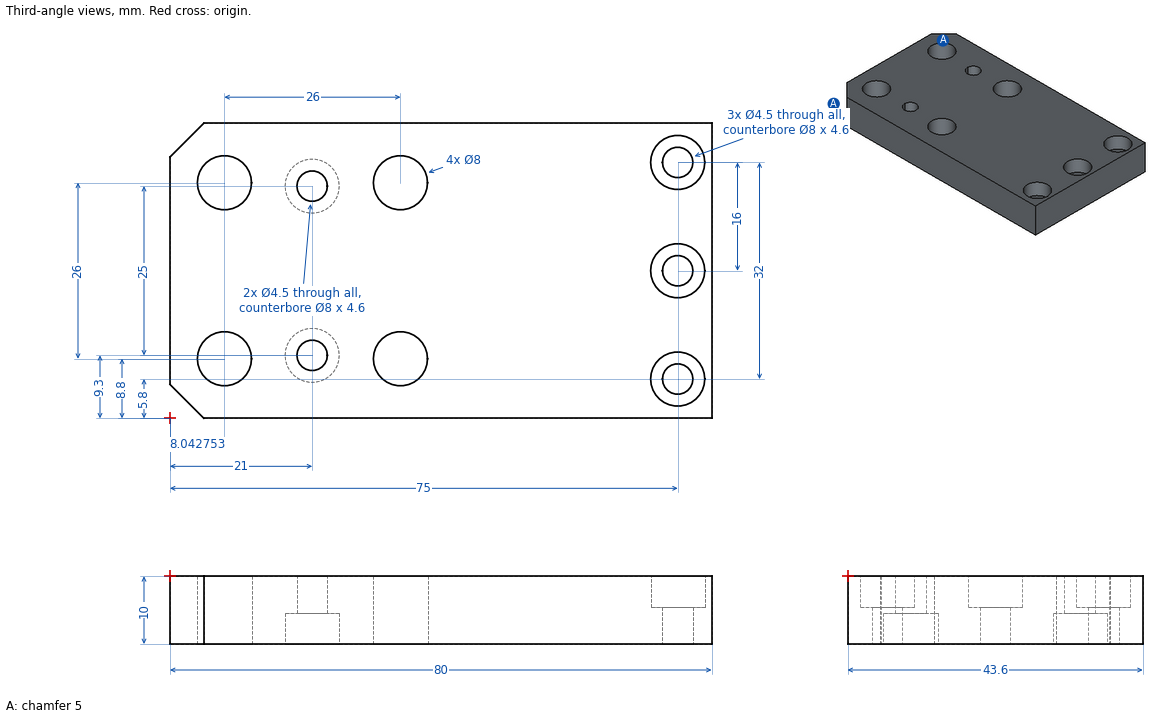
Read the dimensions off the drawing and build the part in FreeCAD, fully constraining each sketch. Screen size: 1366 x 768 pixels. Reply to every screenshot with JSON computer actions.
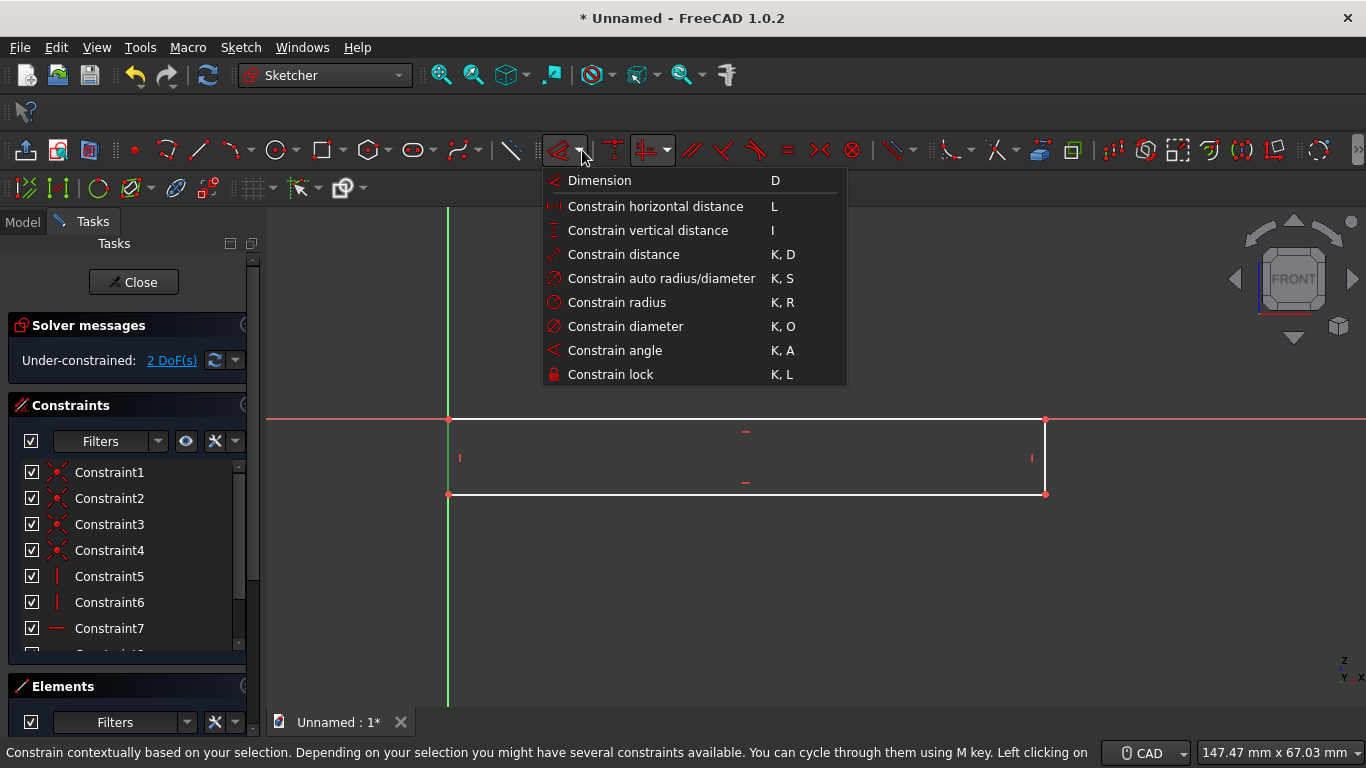
{"action": "left_click", "coordinate": [695, 230]}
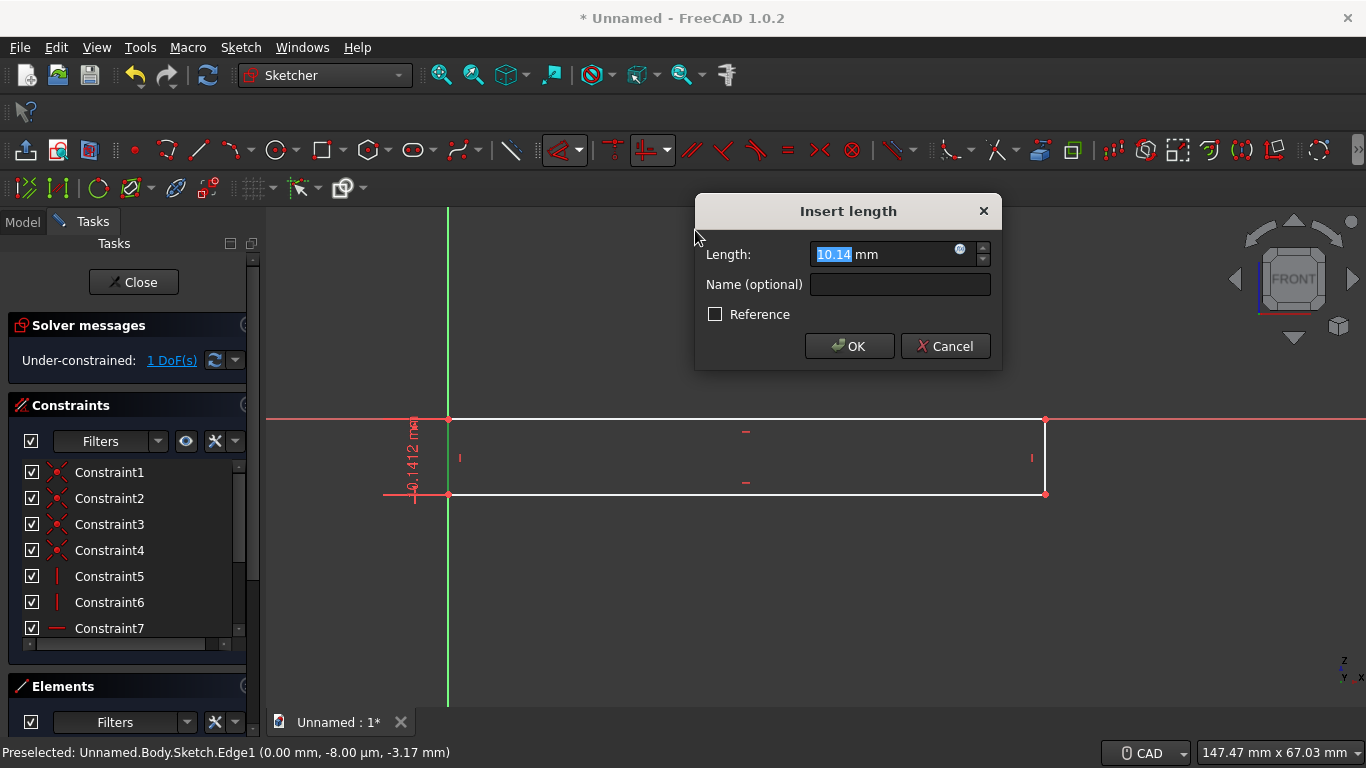
{"action": "type", "text": "10"}
{"action": "key", "text": "Return"}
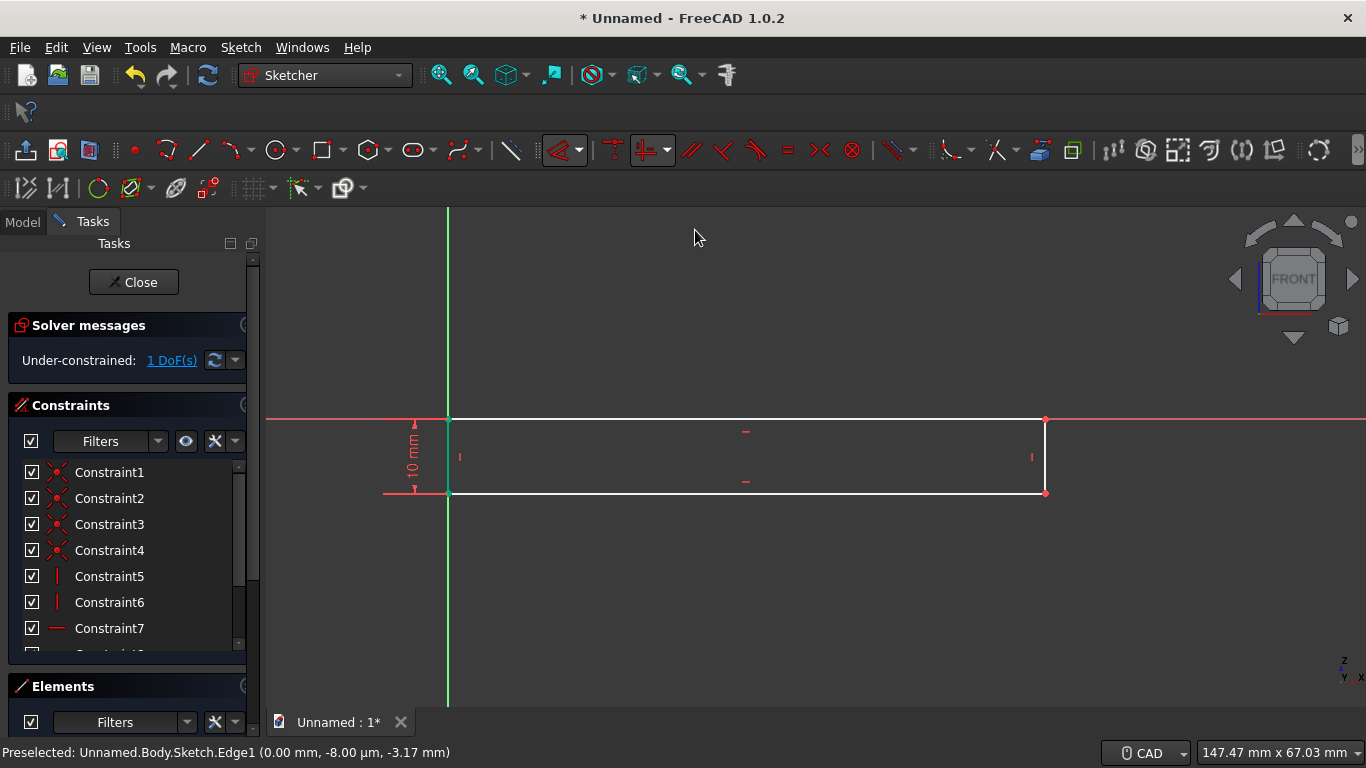
{"action": "left_click", "coordinate": [627, 494]}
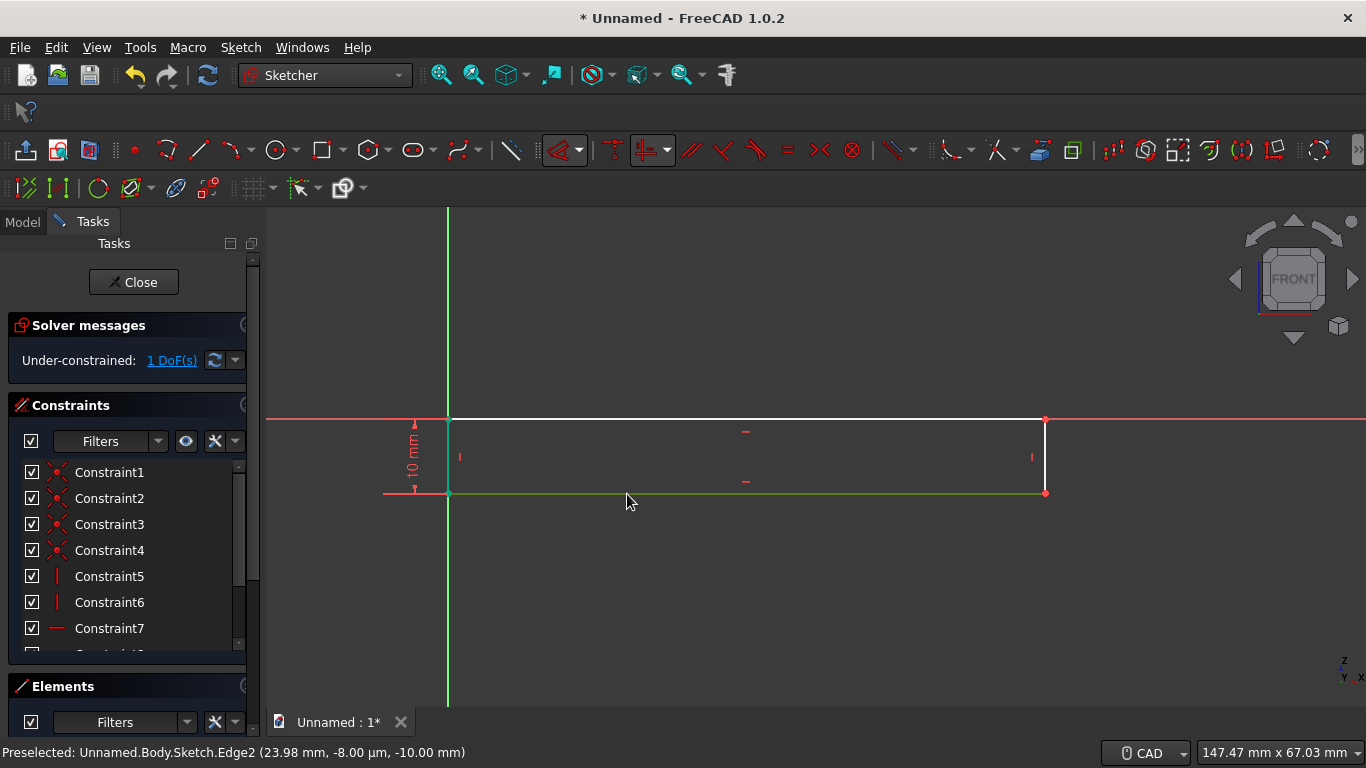
{"action": "key", "text": "l"}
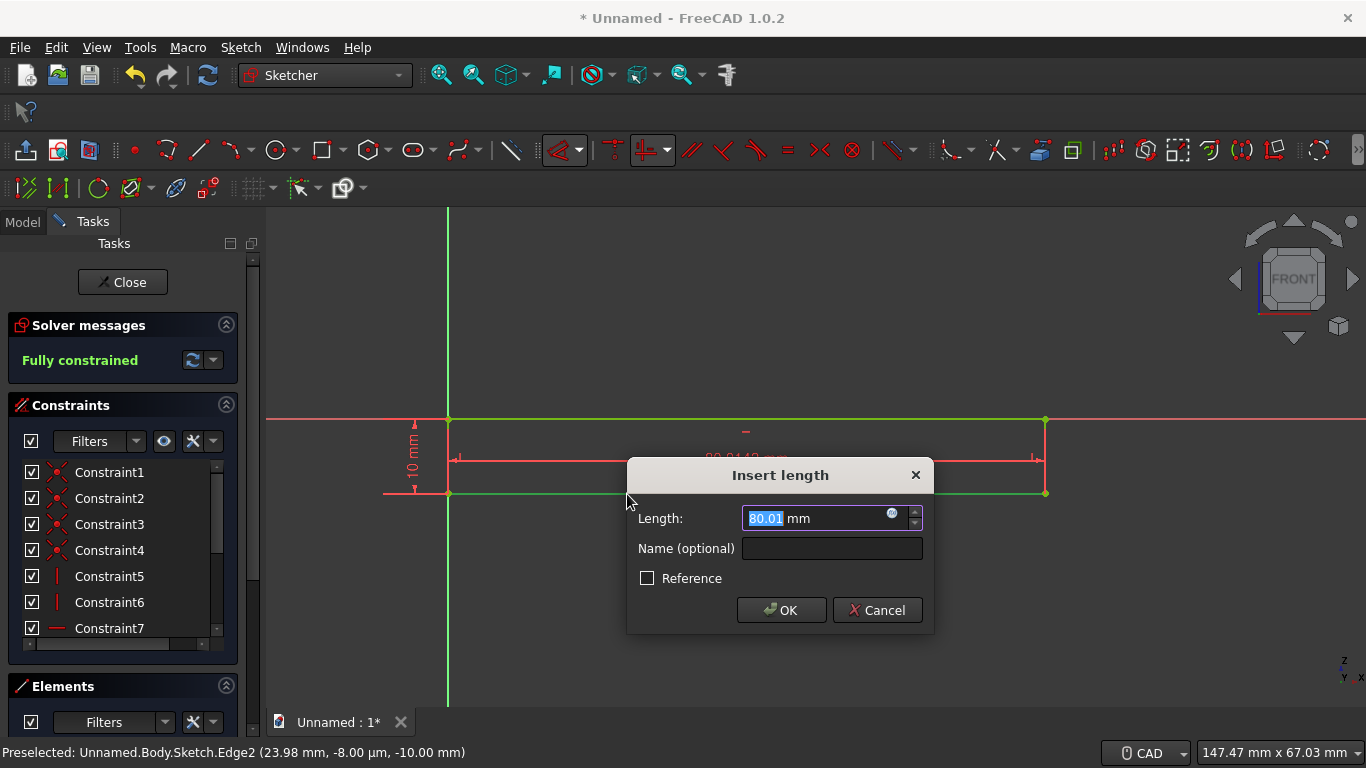
{"action": "type", "text": "80"}
{"action": "key", "text": "Return"}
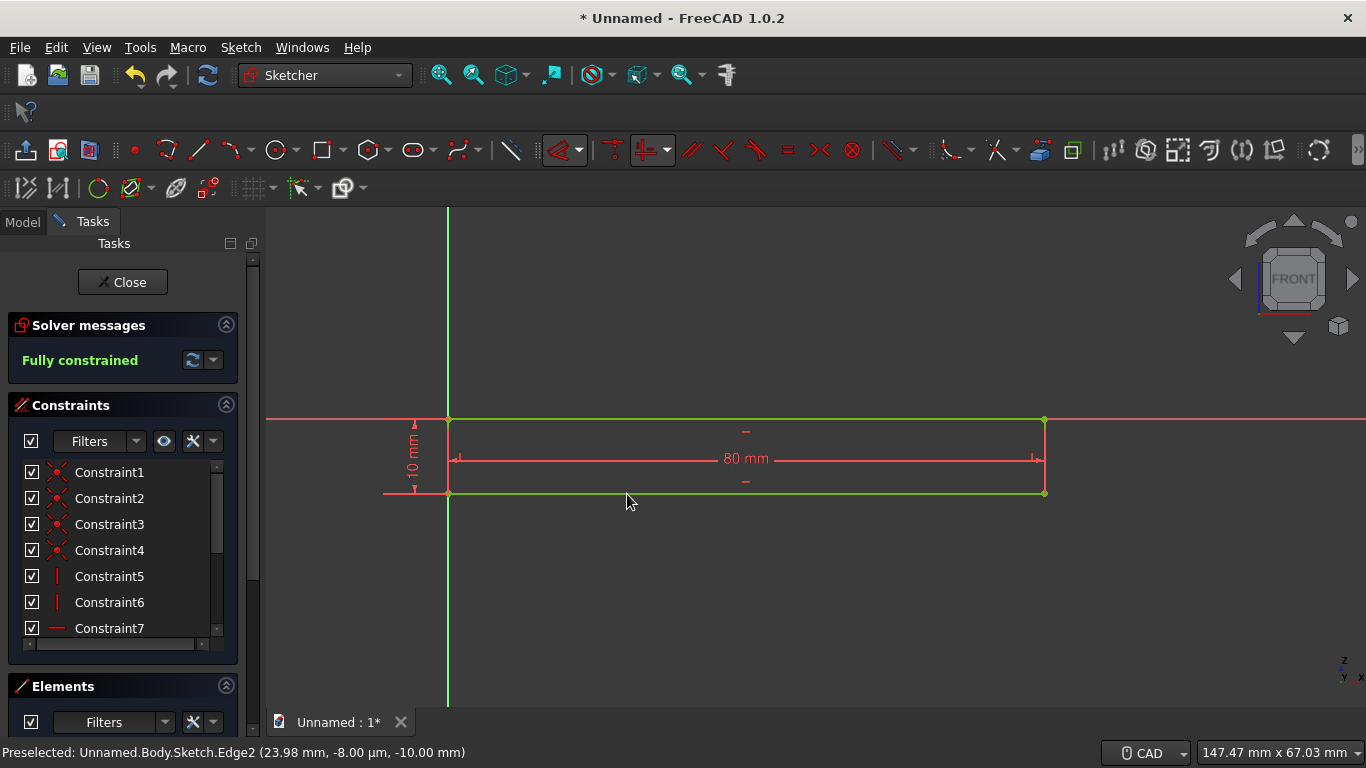
{"action": "left_click", "coordinate": [123, 282]}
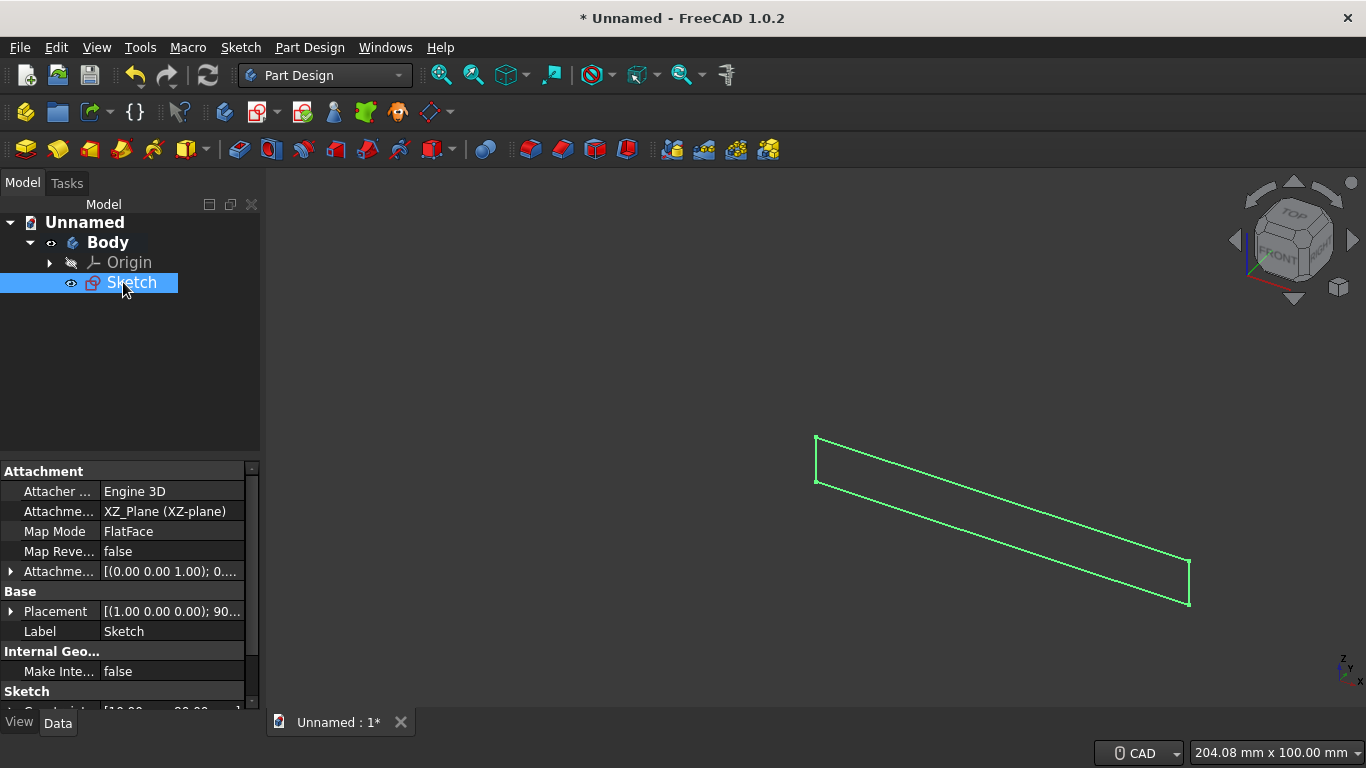
{"action": "left_click", "coordinate": [26, 150]}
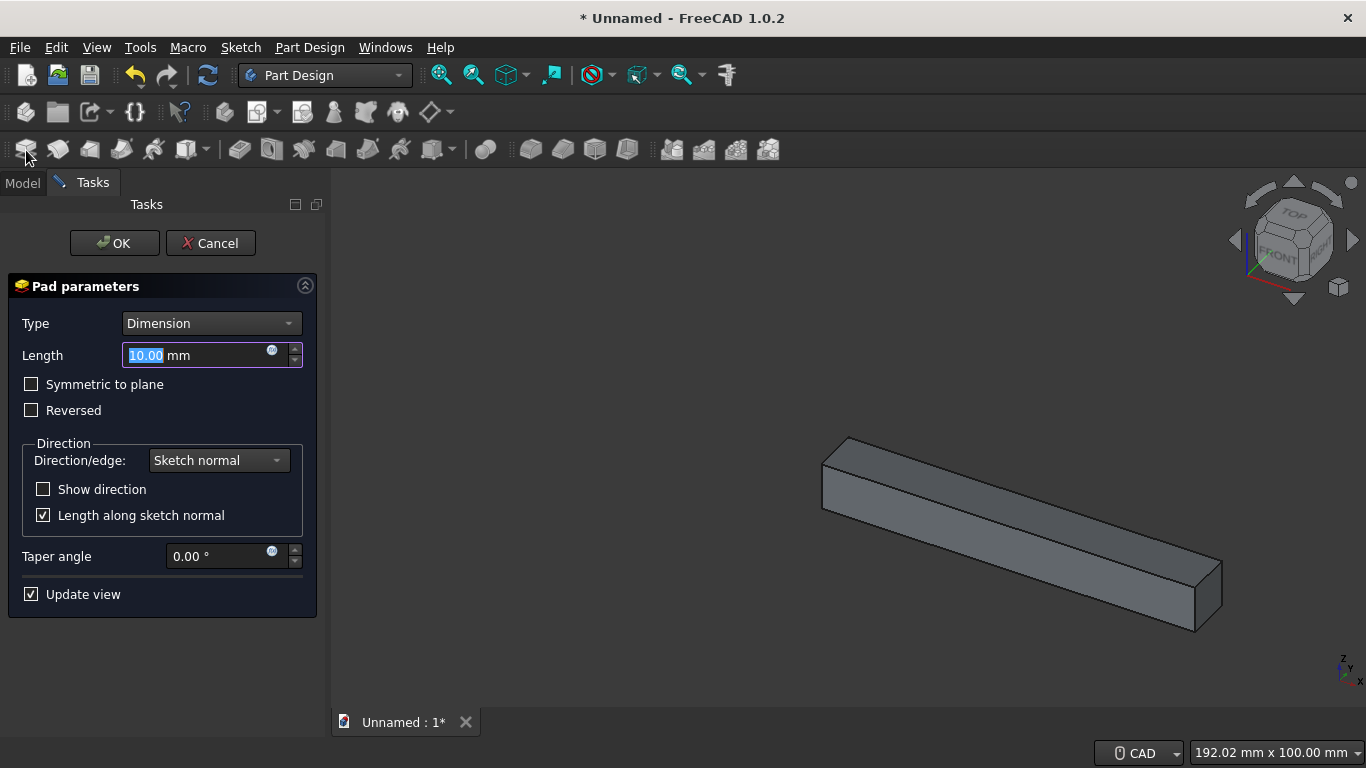
{"action": "type", "text": "43.6"}
{"action": "key", "text": "Tab"}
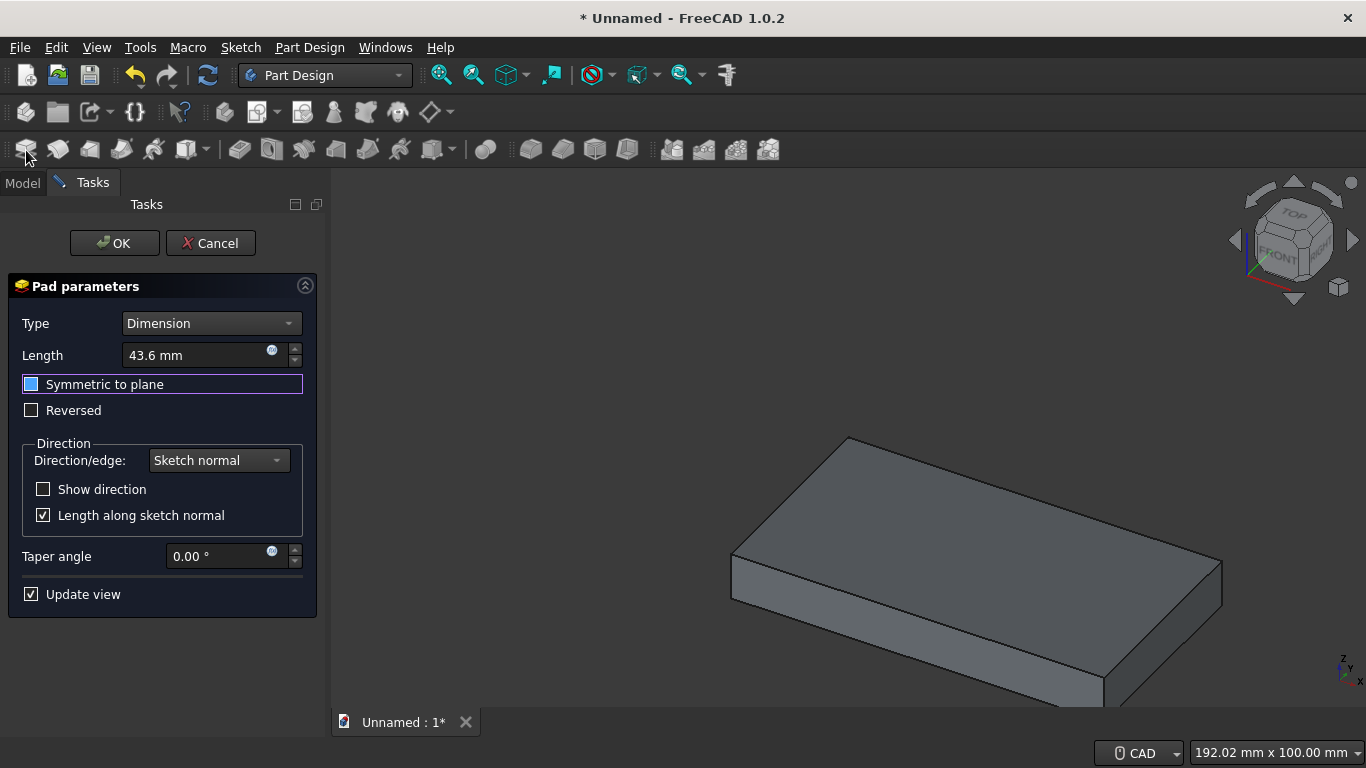
{"action": "left_click", "coordinate": [30, 410]}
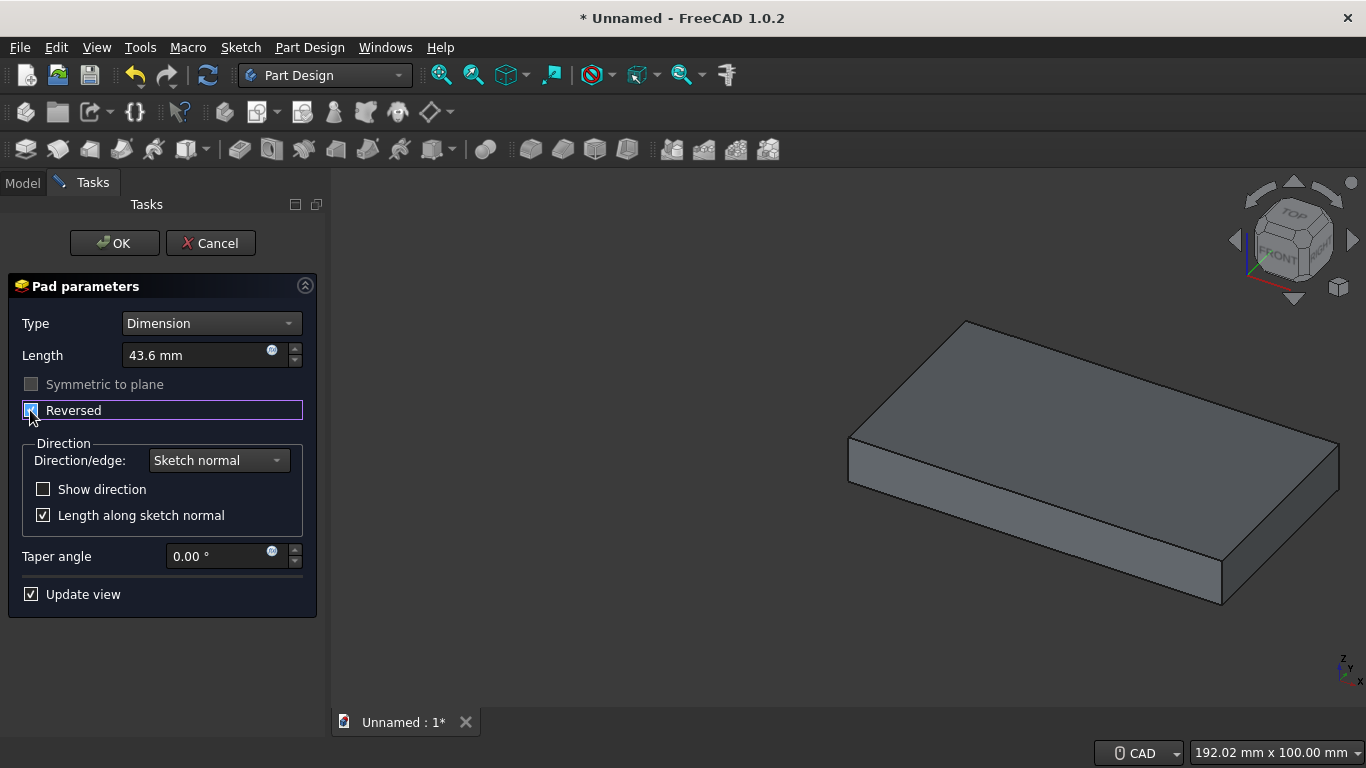
{"action": "left_click", "coordinate": [115, 243]}